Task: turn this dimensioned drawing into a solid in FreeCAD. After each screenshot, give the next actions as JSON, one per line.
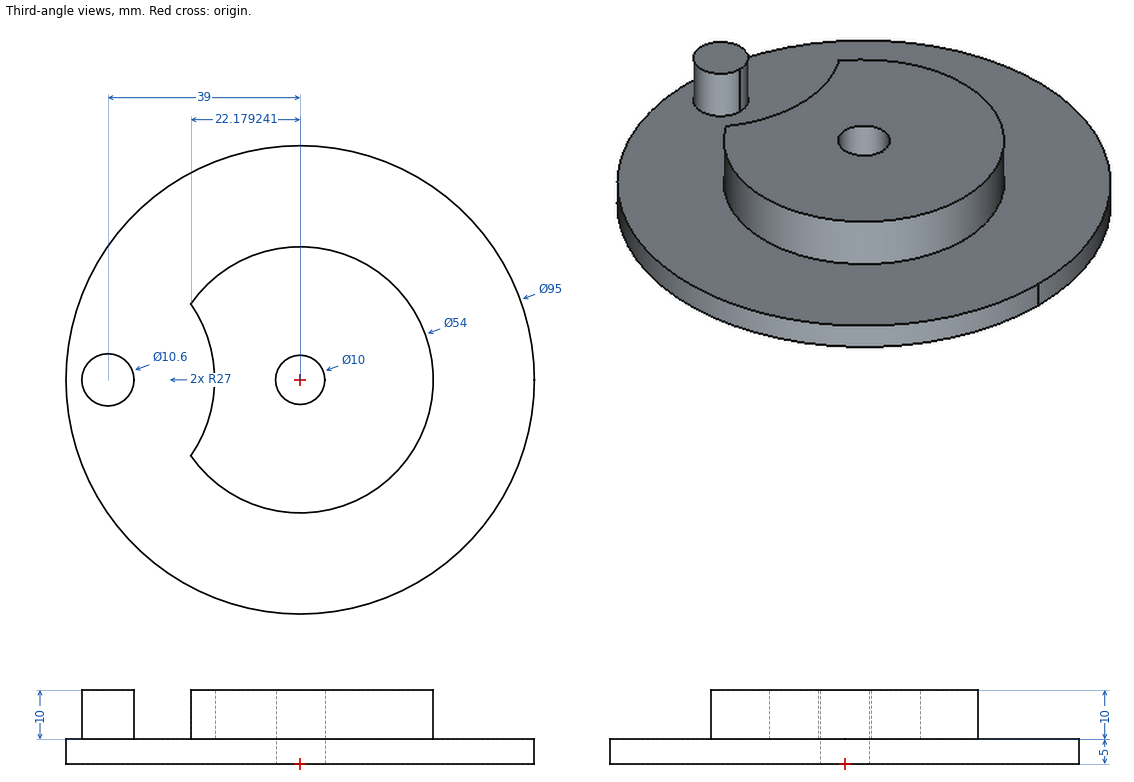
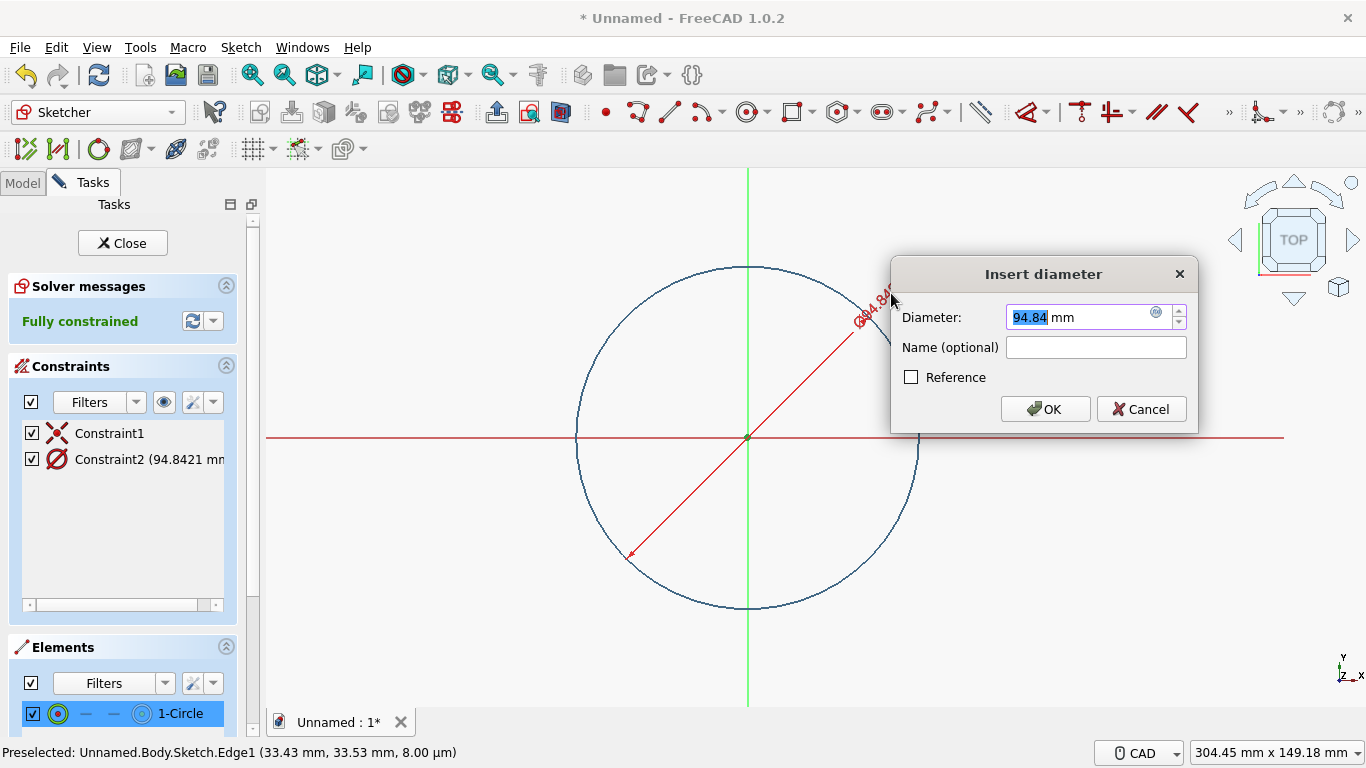
{"action": "type", "text": "95"}
{"action": "key", "text": "Return"}
{"action": "key", "text": "Escape"}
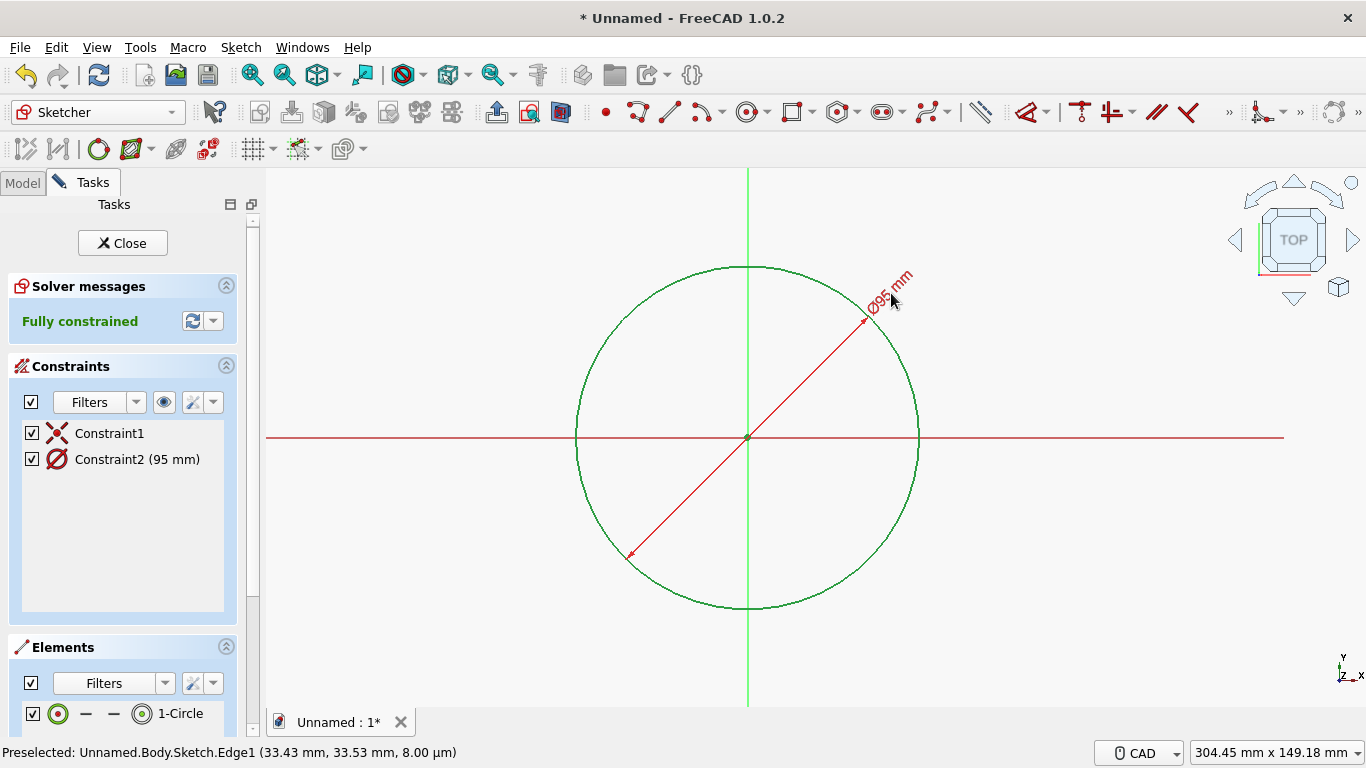
{"action": "left_click", "coordinate": [123, 243]}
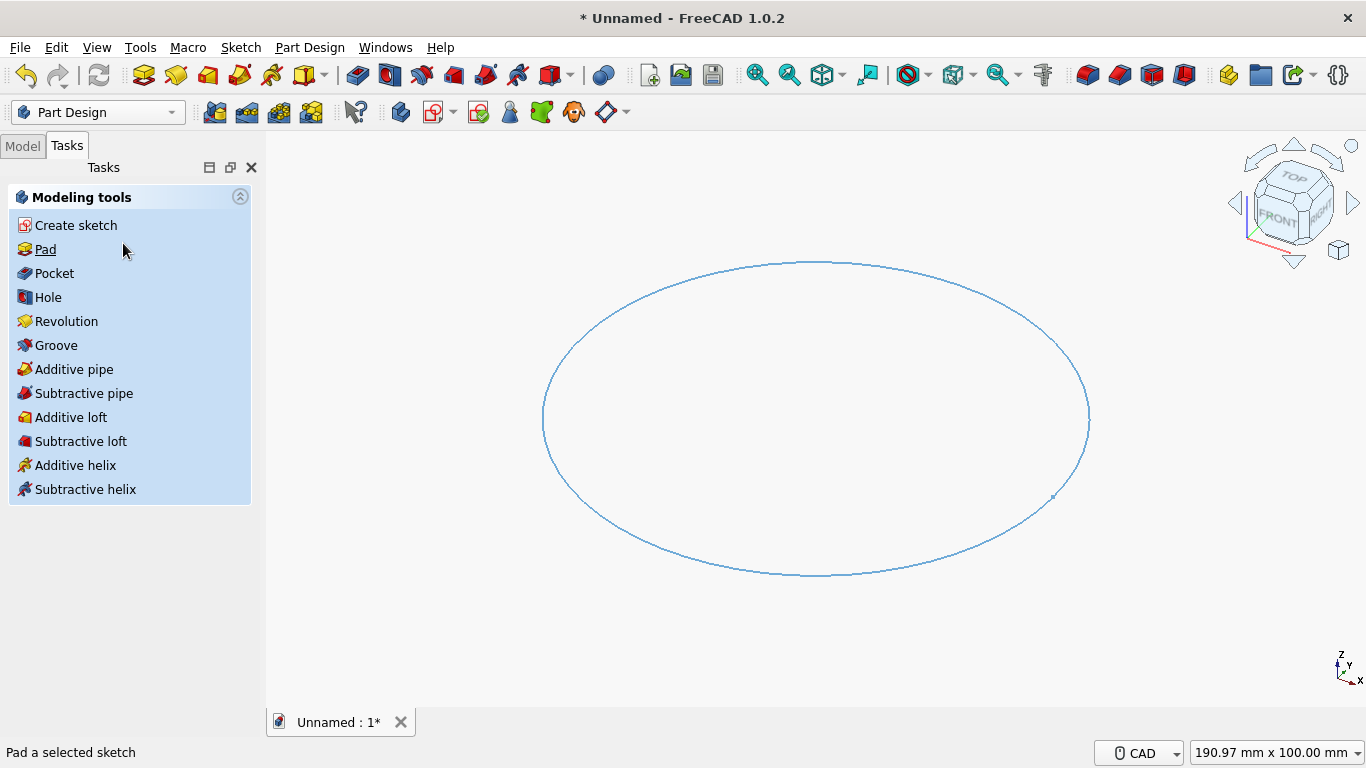
{"action": "left_click", "coordinate": [144, 76]}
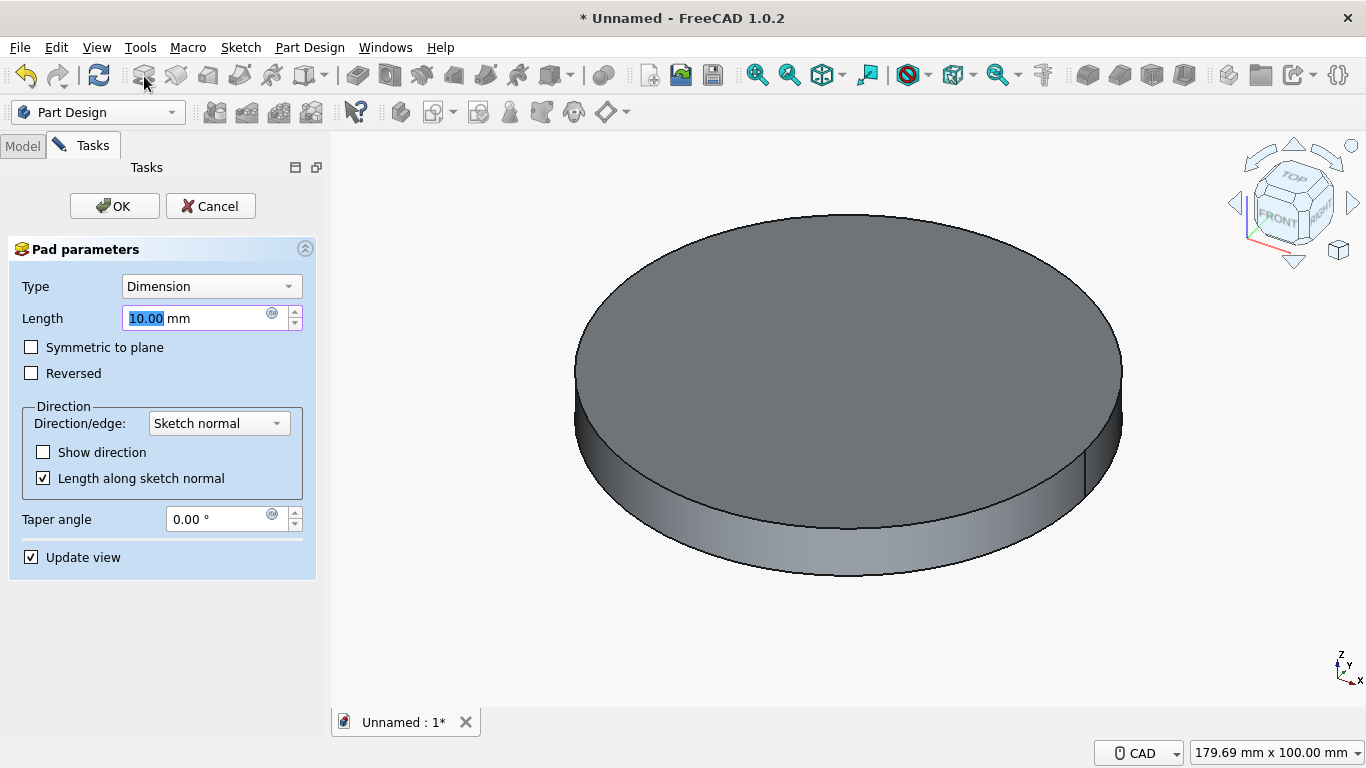
{"action": "type", "text": "5"}
{"action": "key", "text": "Tab"}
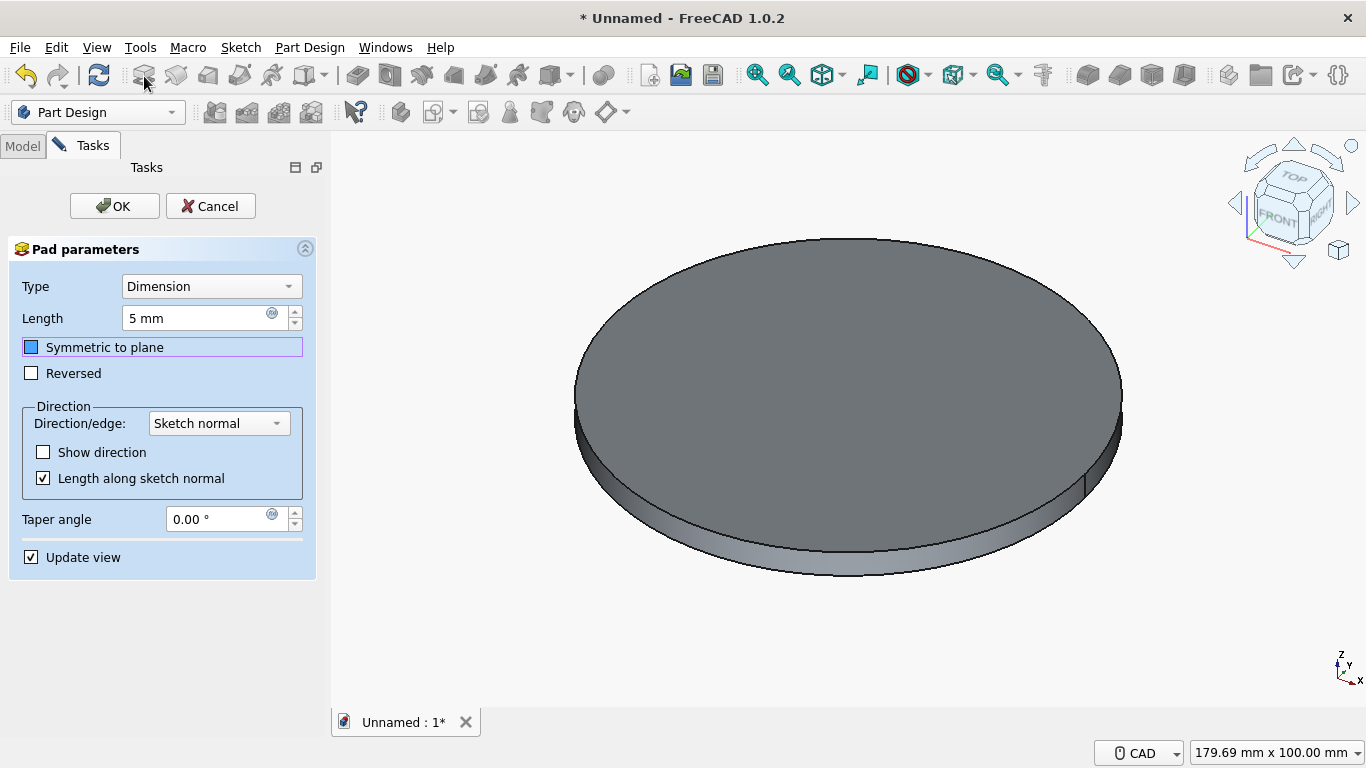
{"action": "left_click", "coordinate": [115, 206]}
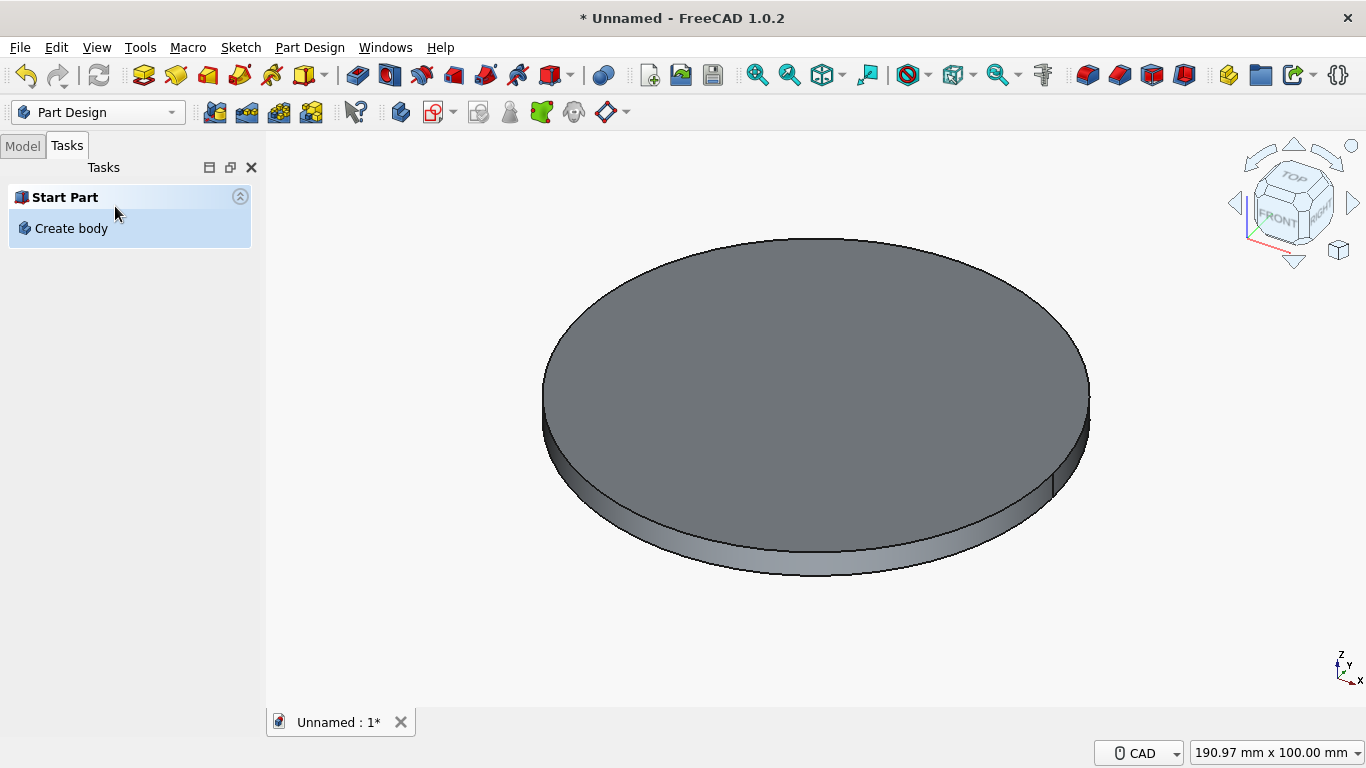
{"action": "left_click", "coordinate": [816, 394]}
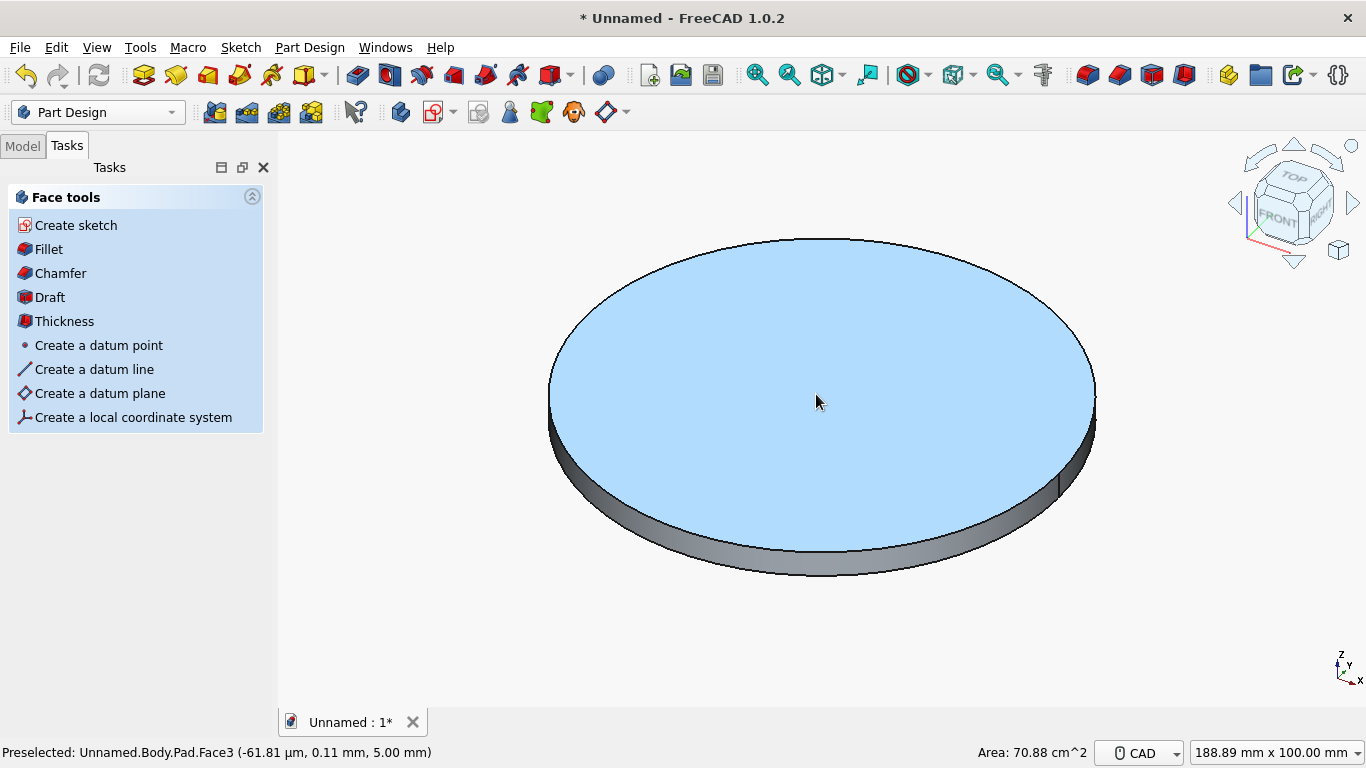
{"action": "left_click", "coordinate": [434, 112]}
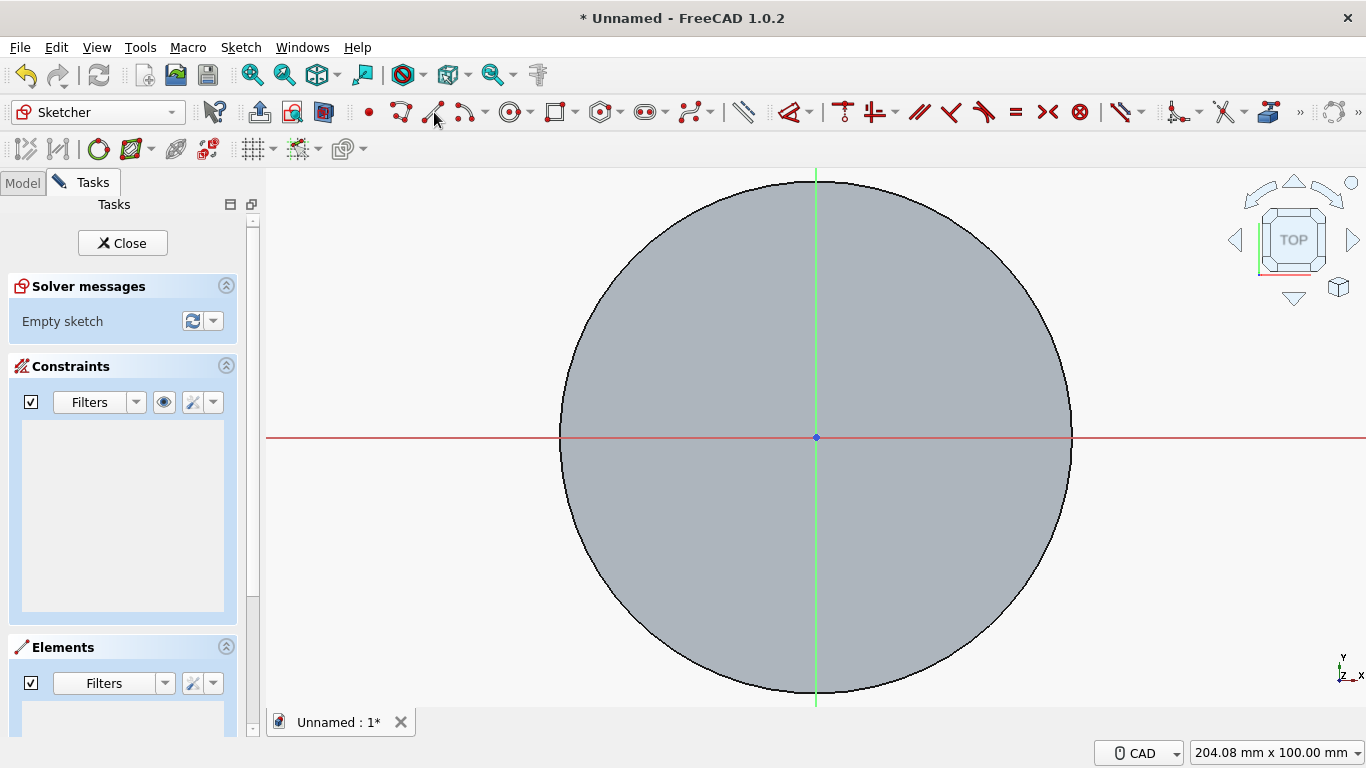
{"action": "scroll", "coordinate": [578, 438], "scroll_direction": "up", "scroll_amount": 9}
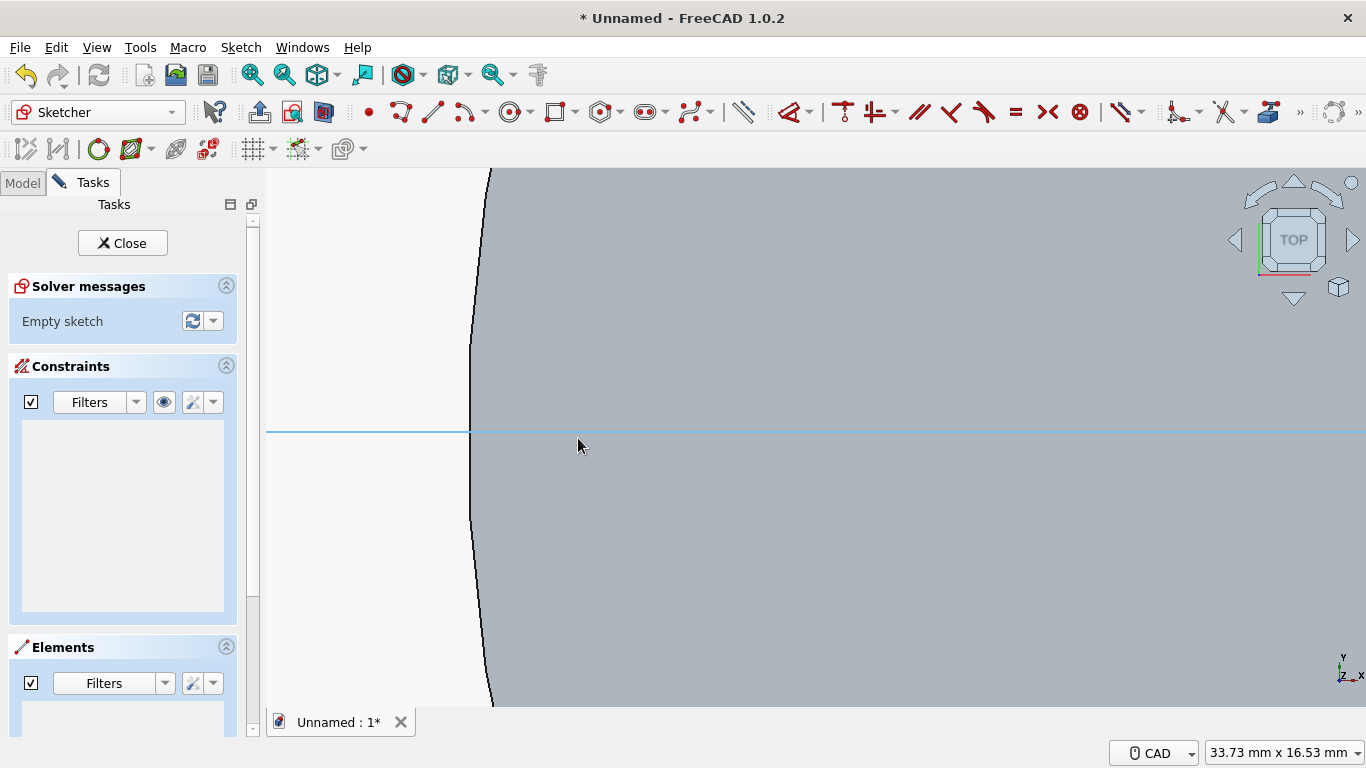
{"action": "key", "text": "g c"}